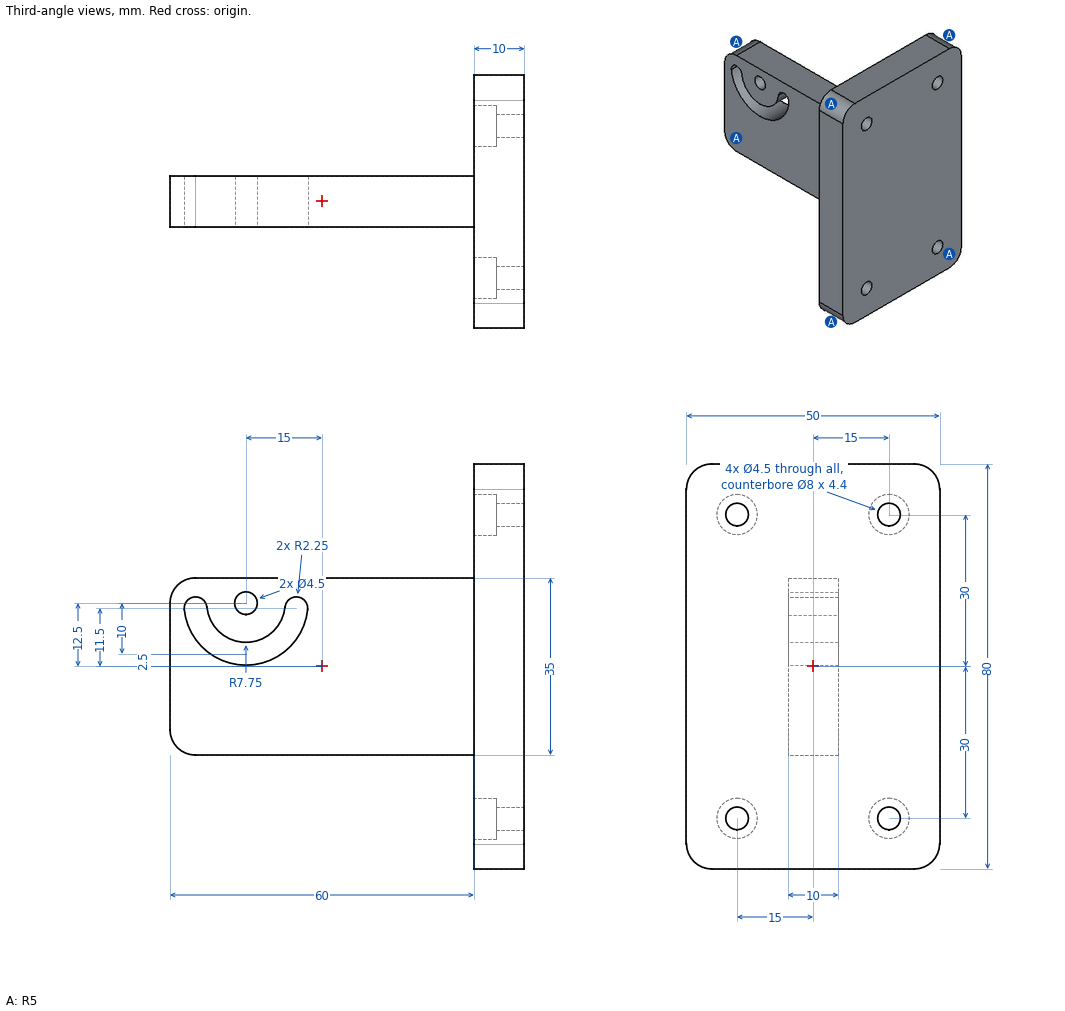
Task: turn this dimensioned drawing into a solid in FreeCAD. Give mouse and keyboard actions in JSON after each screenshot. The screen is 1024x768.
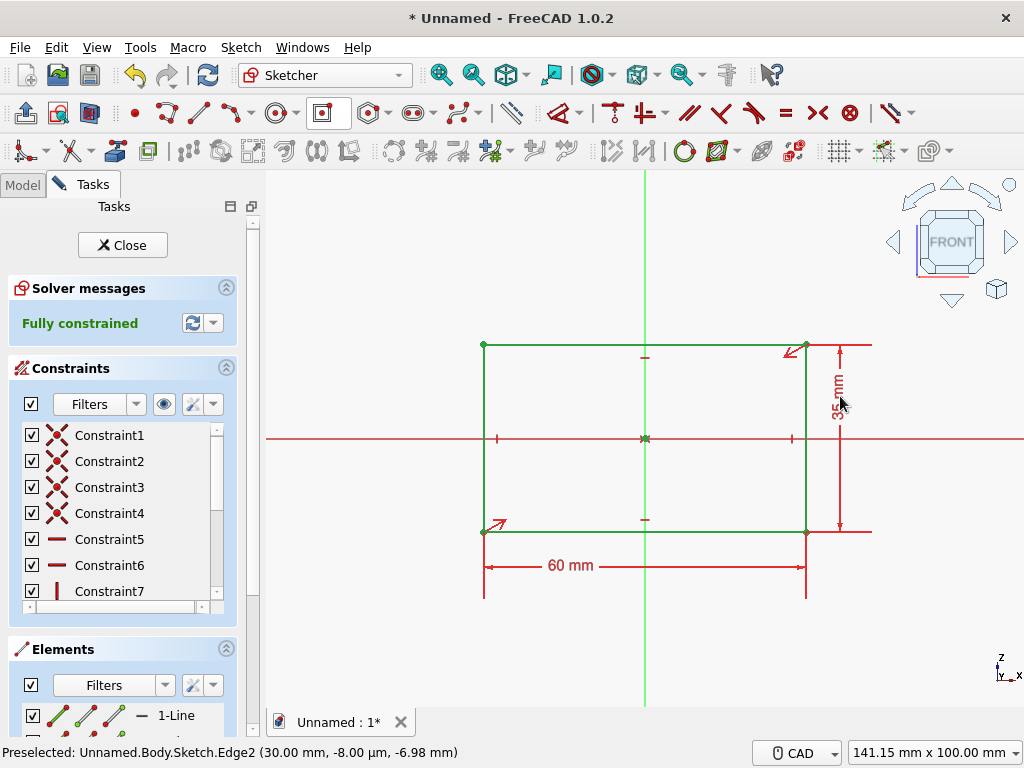
{"action": "left_click", "coordinate": [123, 245]}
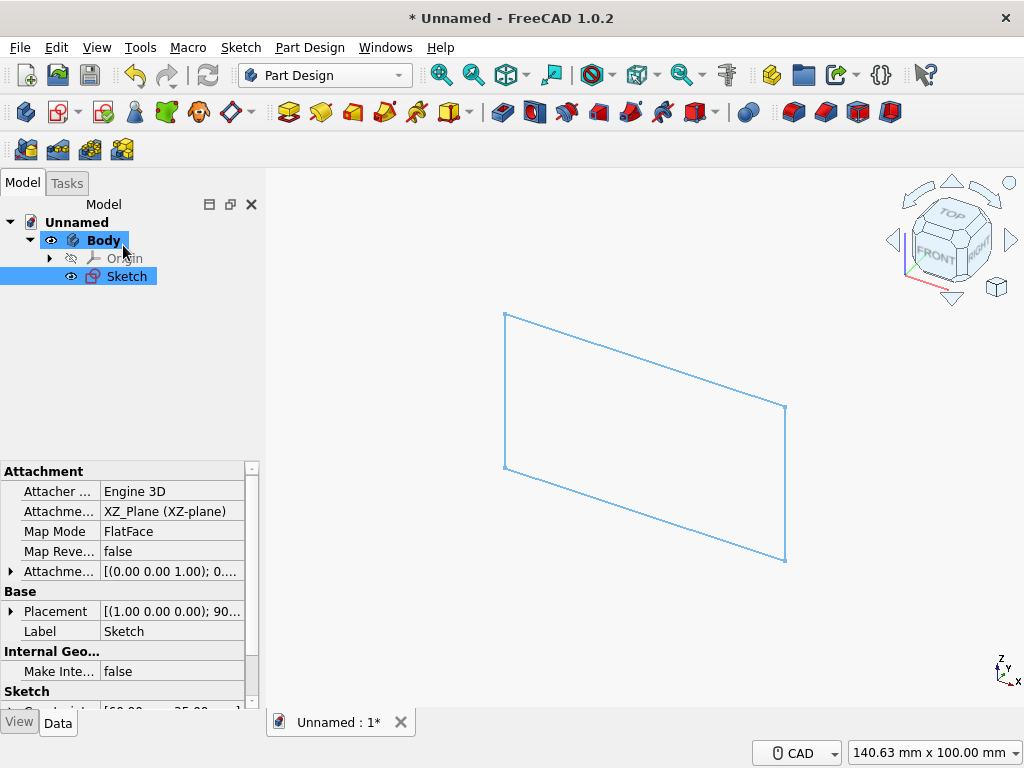
{"action": "left_click", "coordinate": [290, 112]}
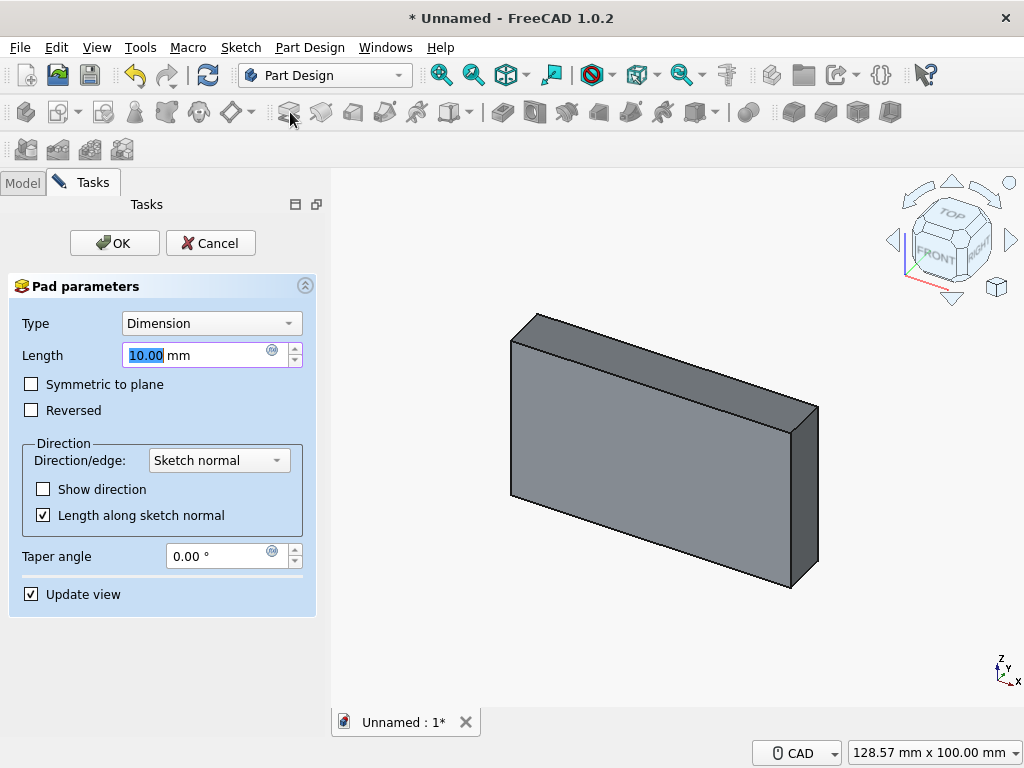
{"action": "type", "text": "10"}
{"action": "key", "text": "Tab"}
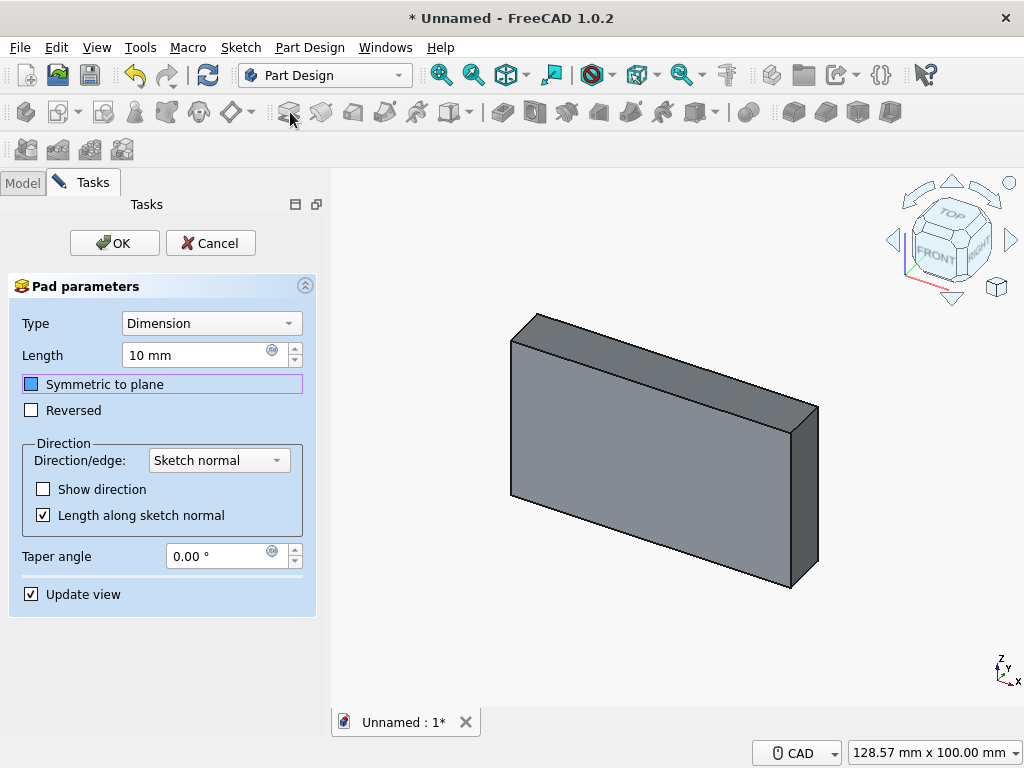
{"action": "left_click", "coordinate": [30, 384]}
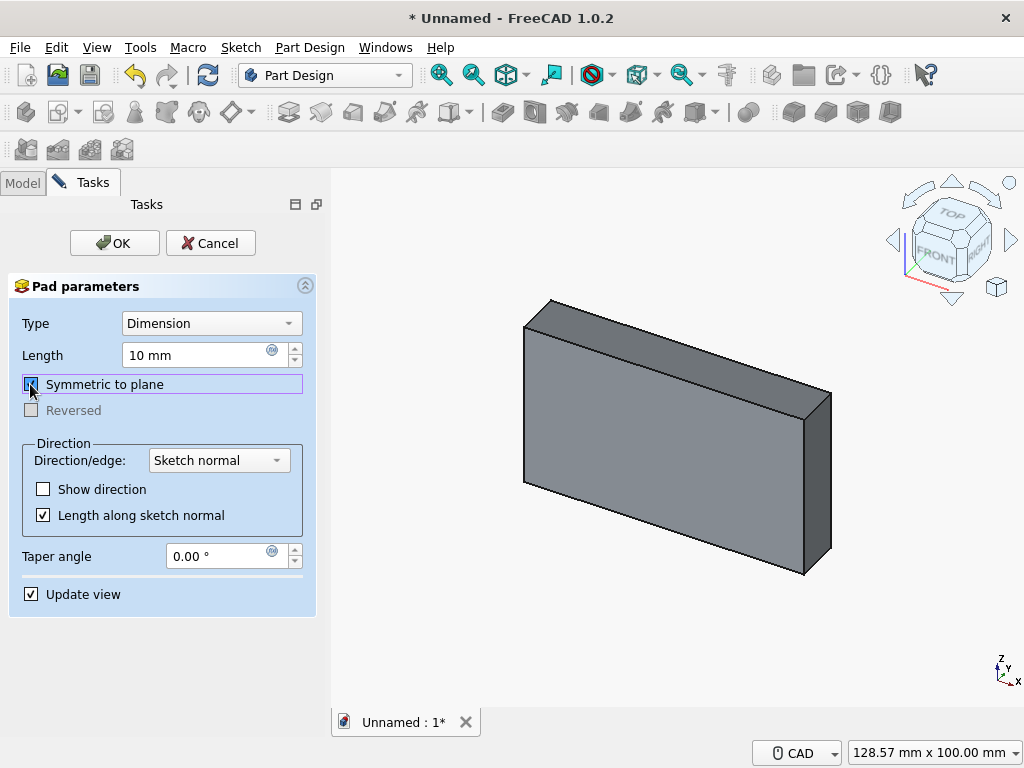
{"action": "left_click", "coordinate": [115, 243]}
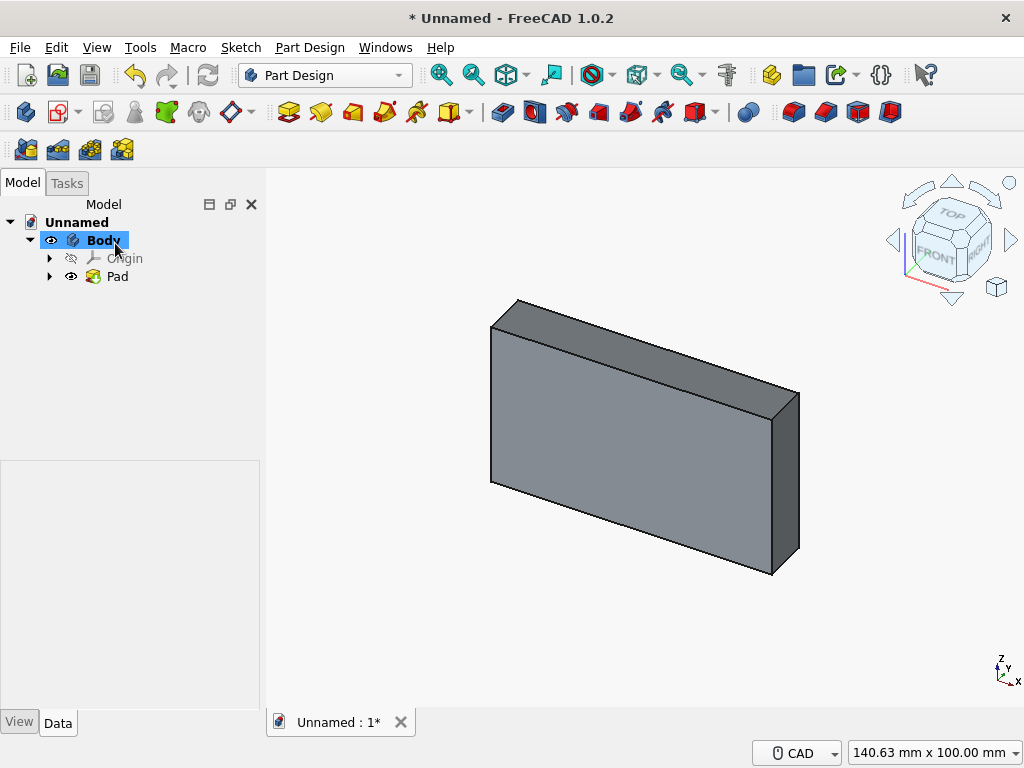
{"action": "left_click", "coordinate": [672, 463]}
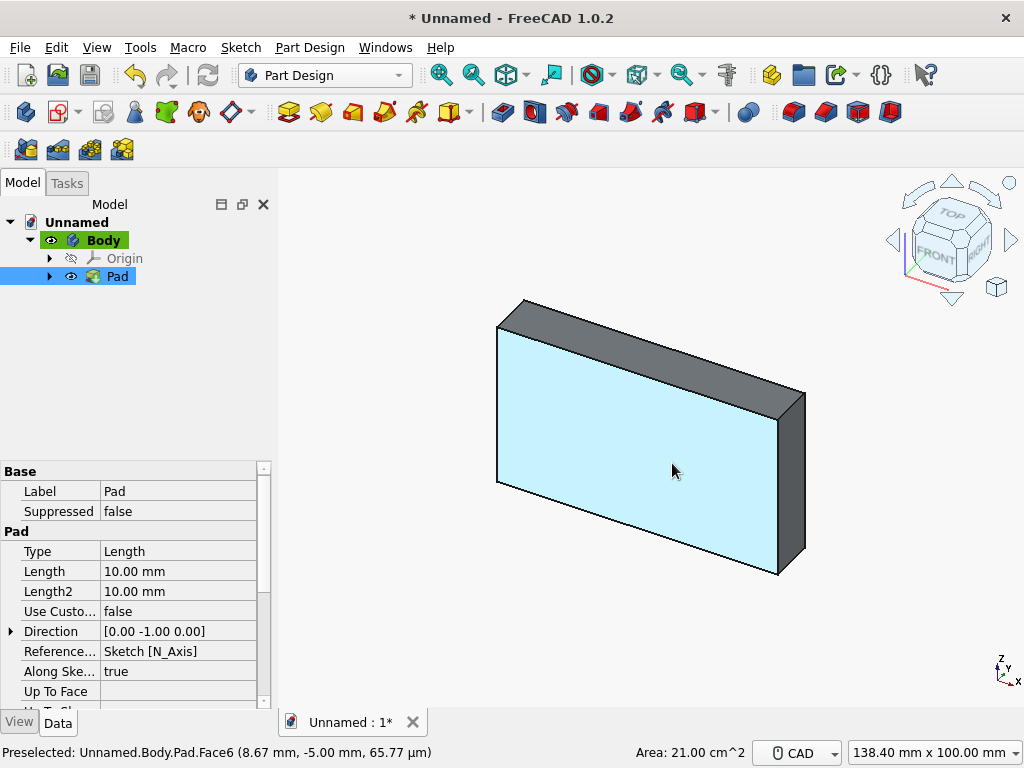
{"action": "left_click", "coordinate": [58, 112]}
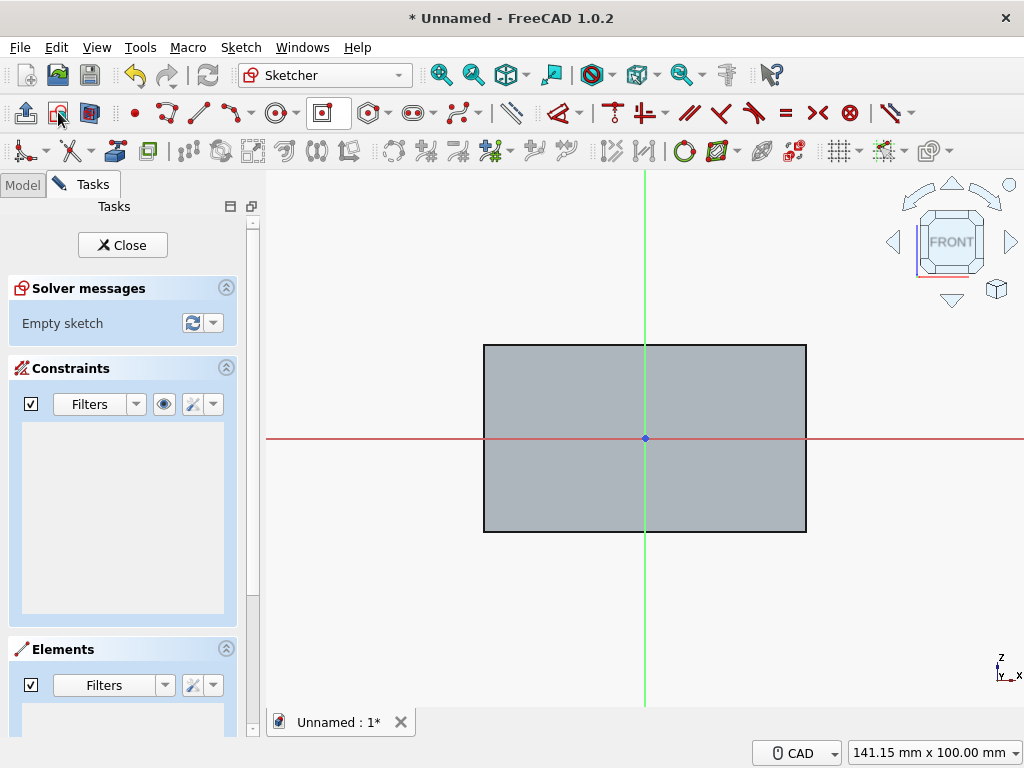
{"action": "scroll", "coordinate": [606, 386], "scroll_direction": "up", "scroll_amount": 7}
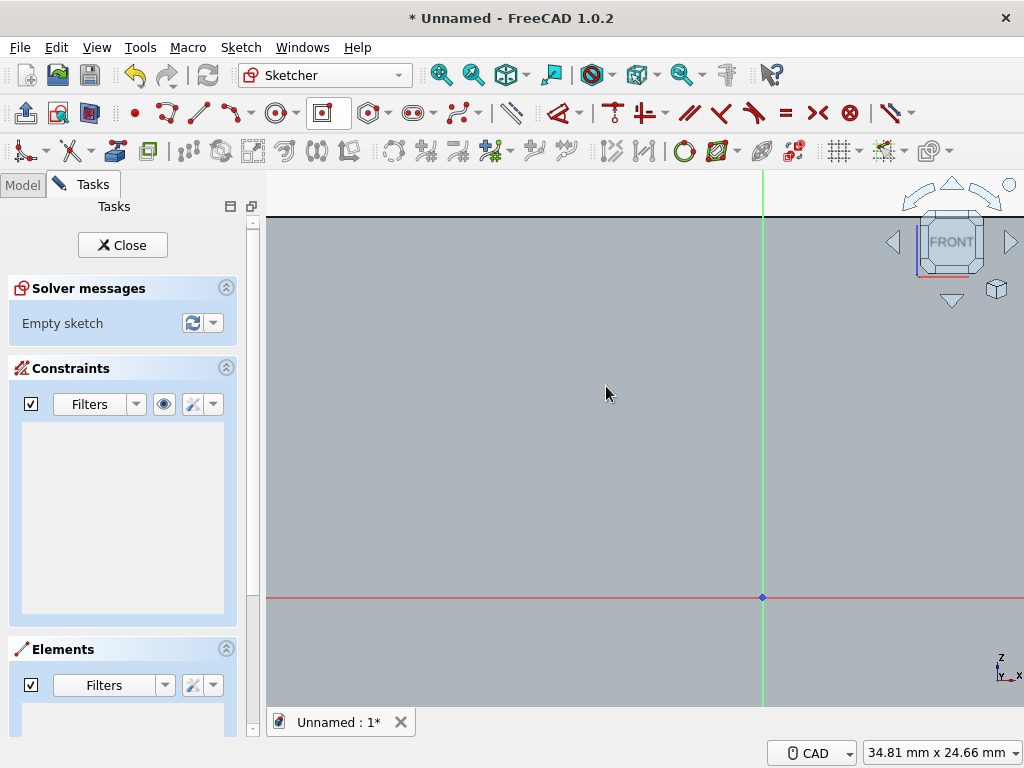
{"action": "left_click", "coordinate": [276, 114]}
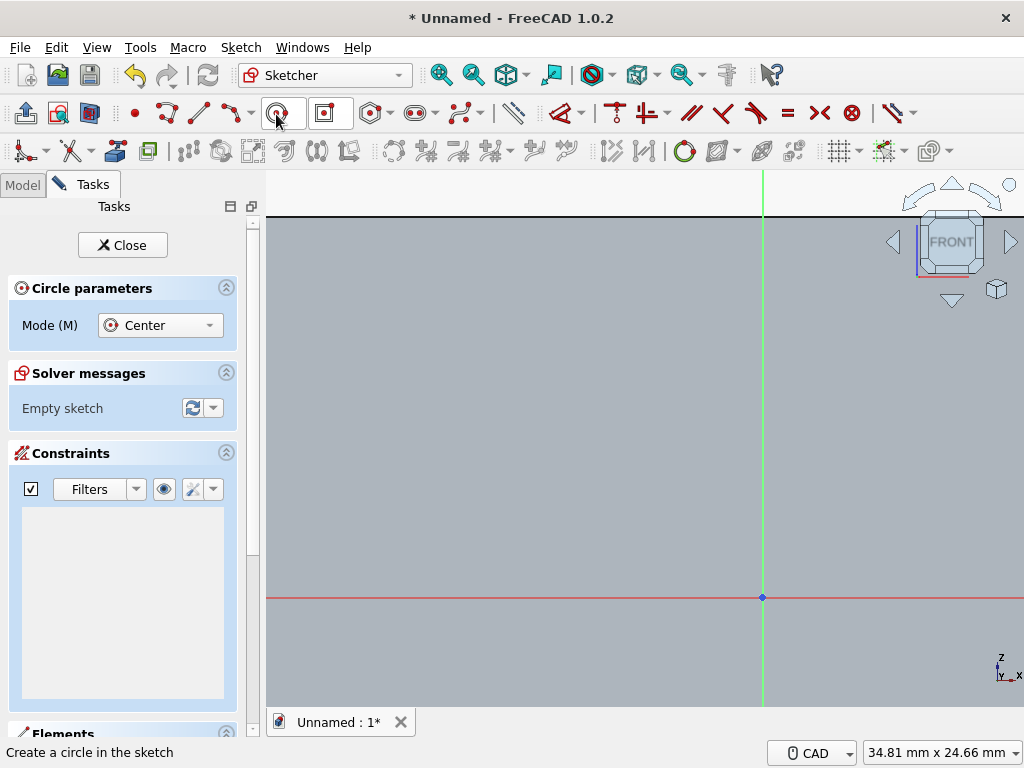
{"action": "left_click", "coordinate": [436, 325]}
{"action": "left_click", "coordinate": [471, 291]}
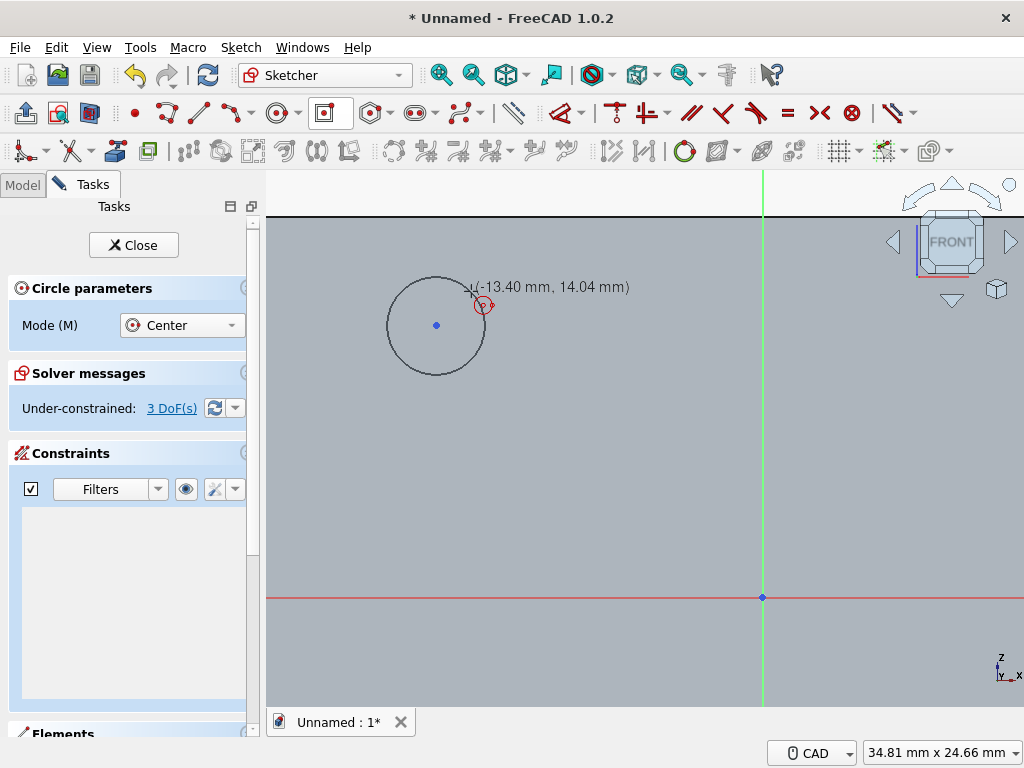
{"action": "left_click", "coordinate": [436, 543]}
{"action": "left_click", "coordinate": [471, 509]}
{"action": "key", "text": "Escape"}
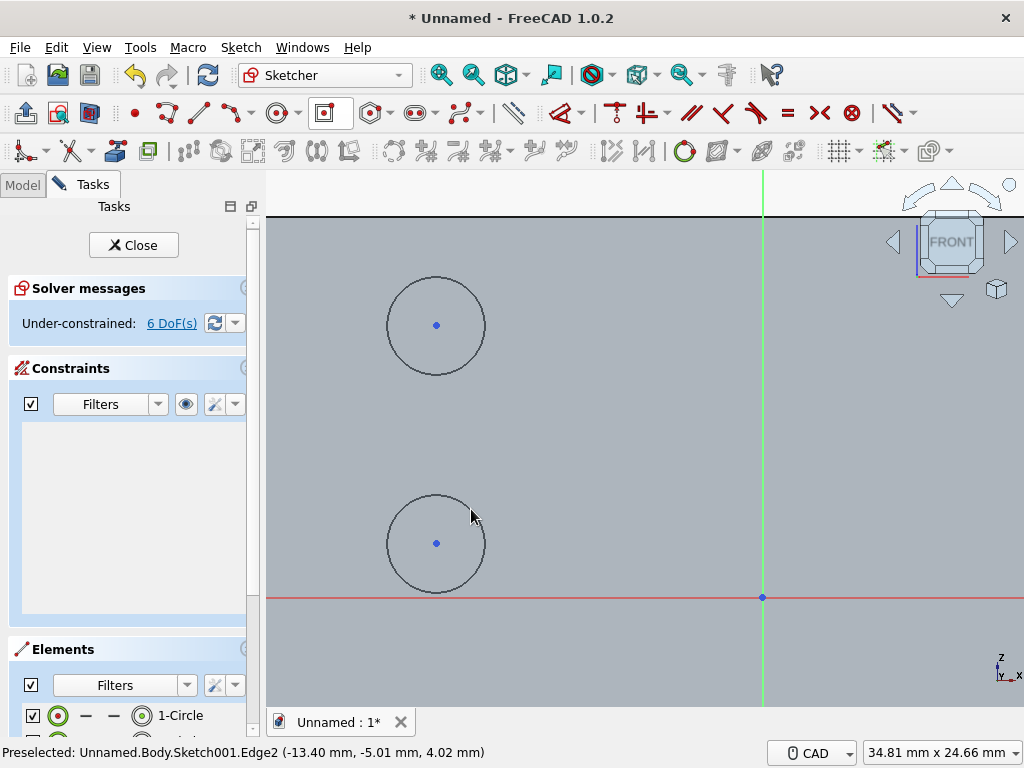
{"action": "left_click", "coordinate": [470, 291]}